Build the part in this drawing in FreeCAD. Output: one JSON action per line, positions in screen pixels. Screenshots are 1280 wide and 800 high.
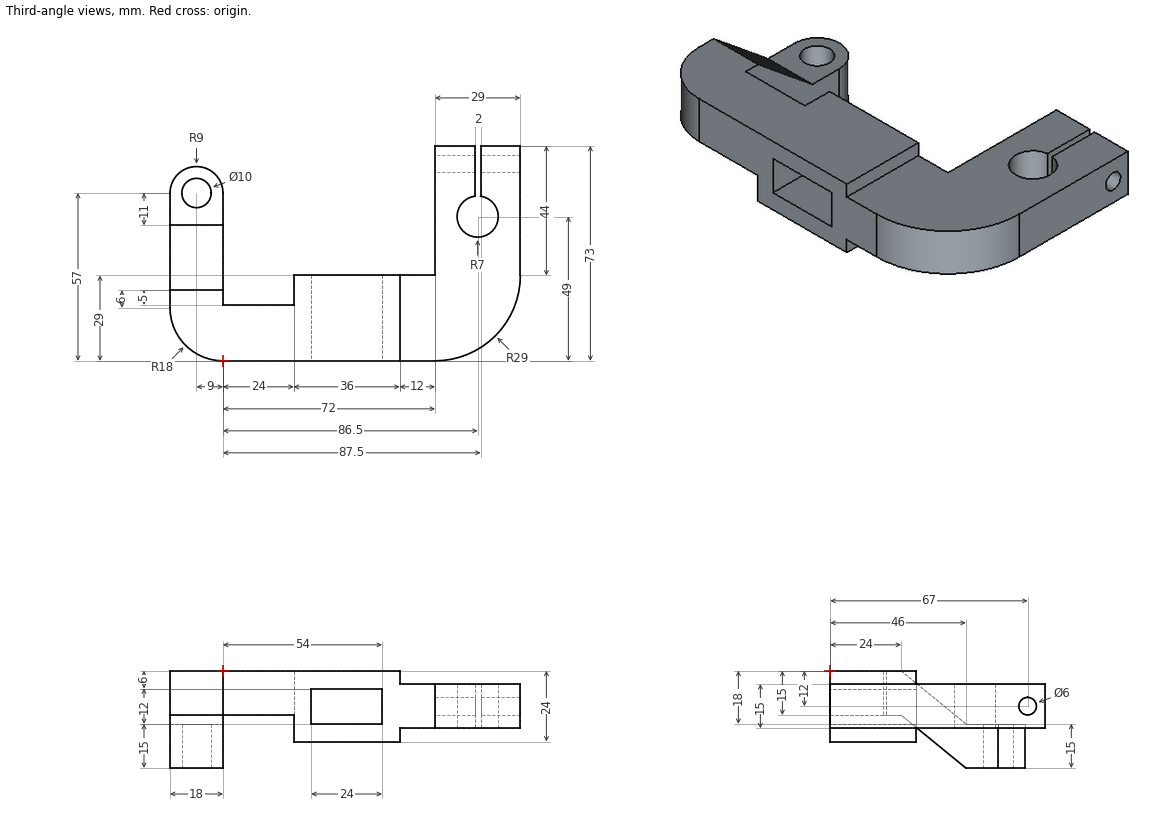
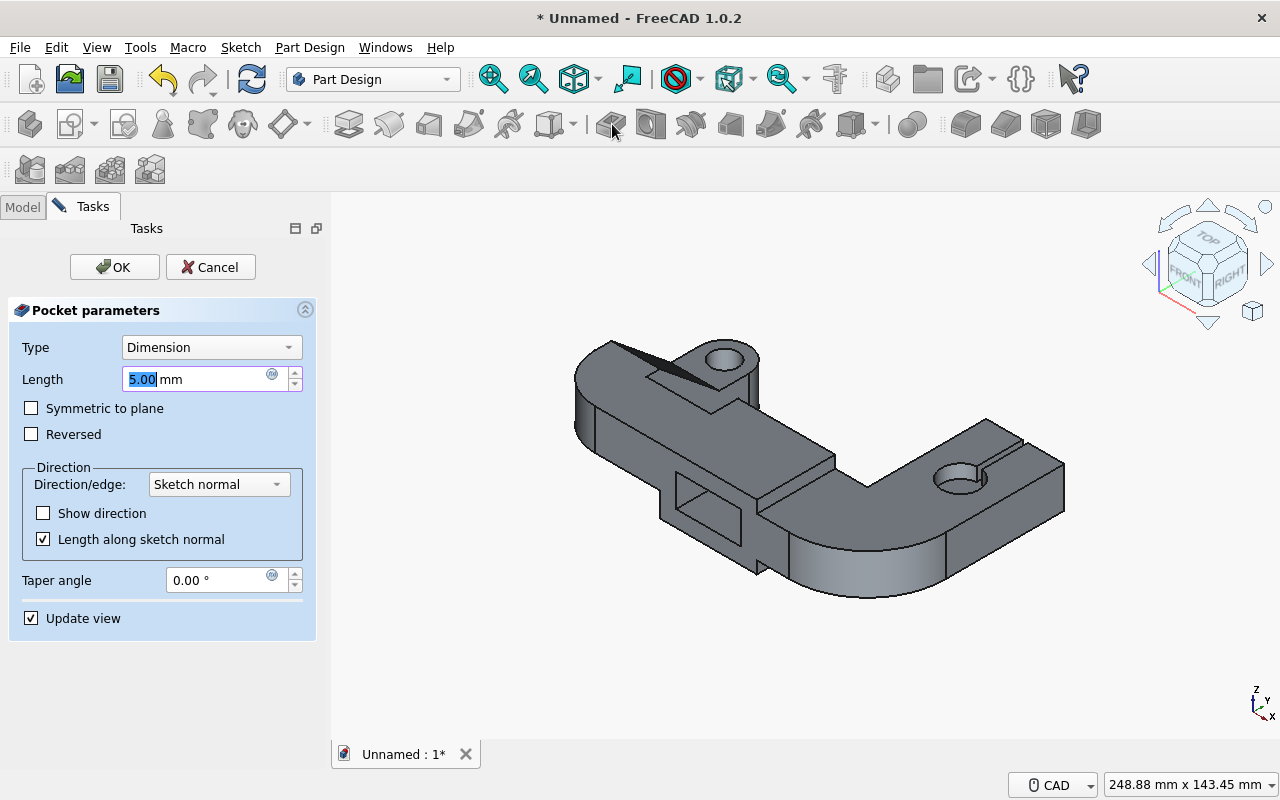
{"action": "type", "text": "15"}
{"action": "key", "text": "Tab"}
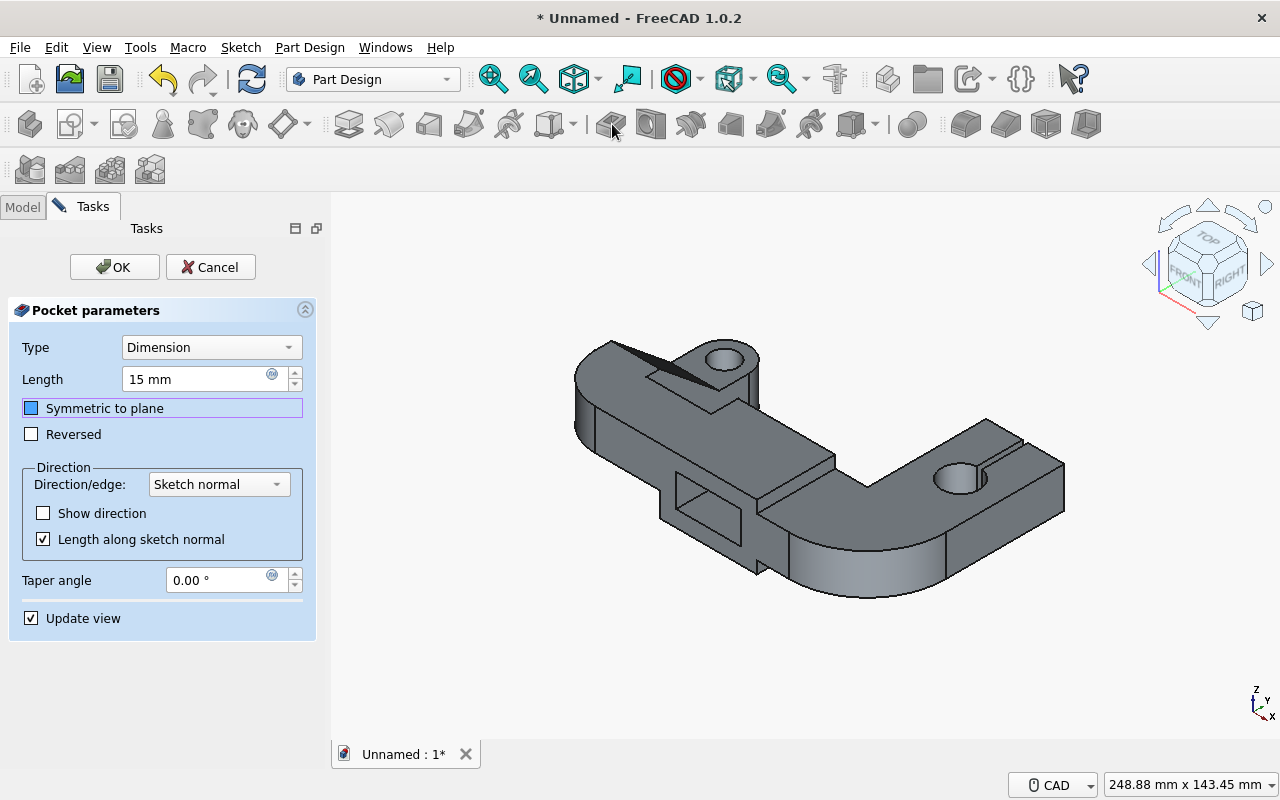
{"action": "left_click", "coordinate": [115, 267]}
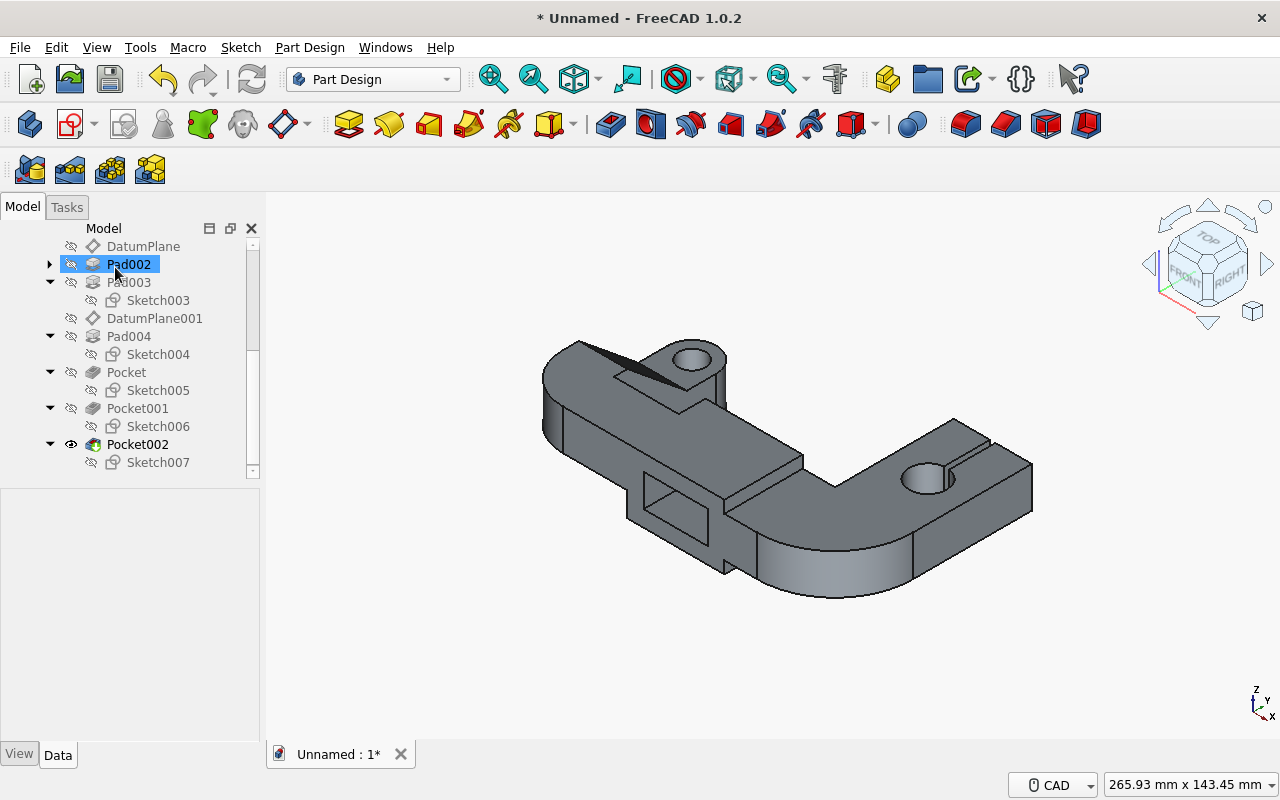
{"action": "key", "text": "6"}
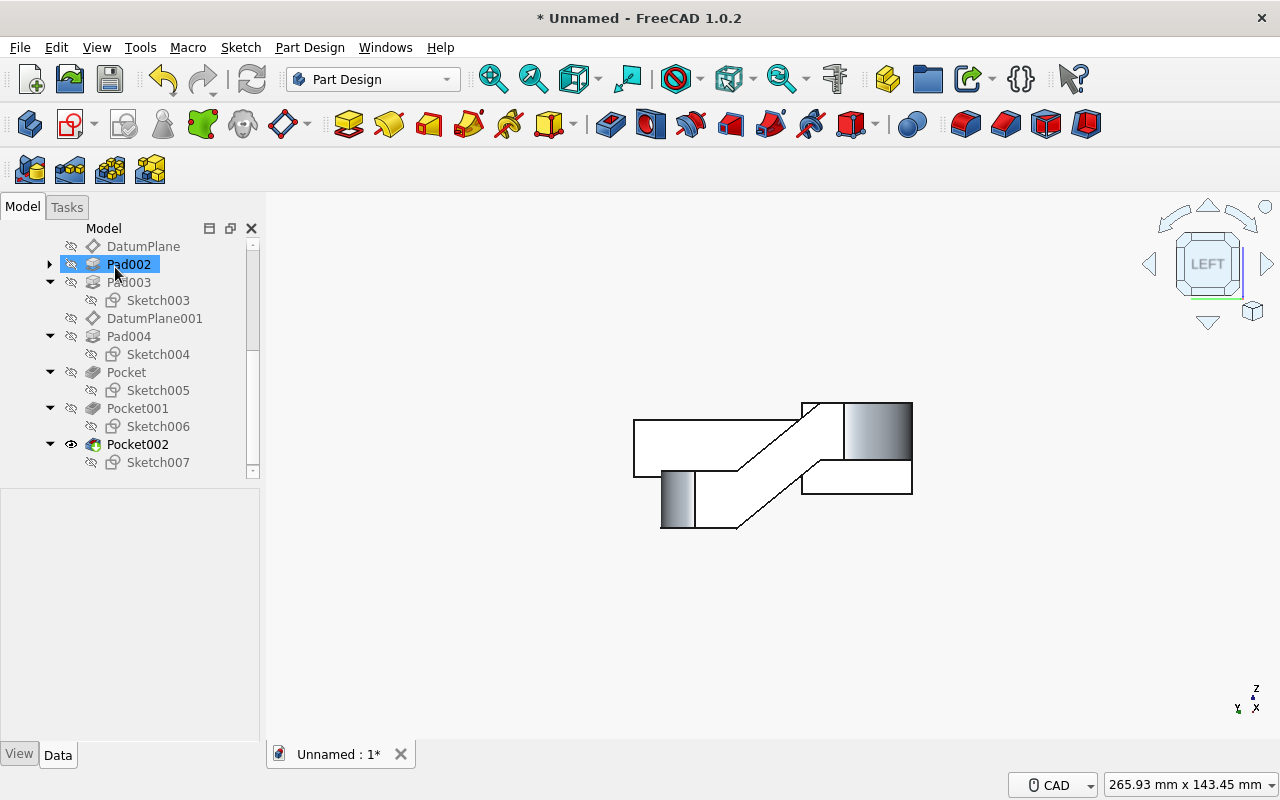
{"action": "left_click", "coordinate": [494, 80]}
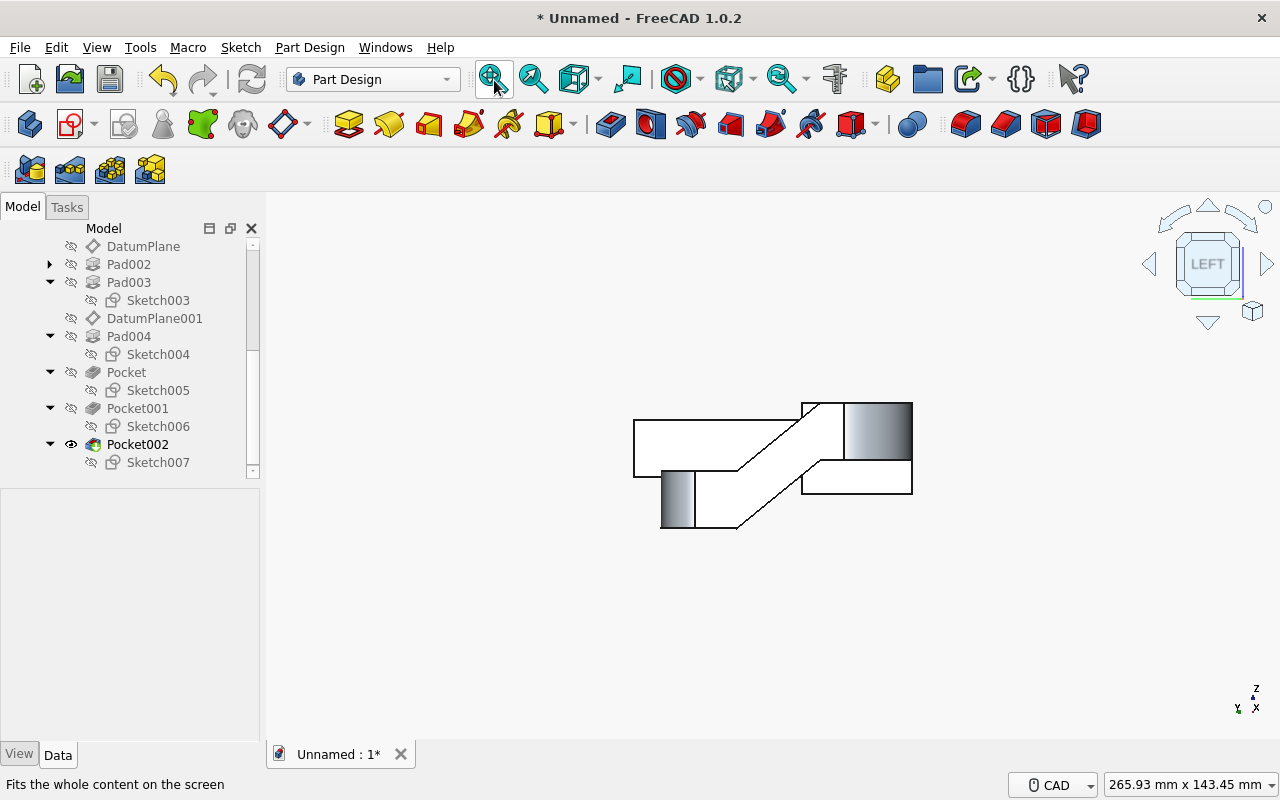
{"action": "left_click", "coordinate": [670, 447]}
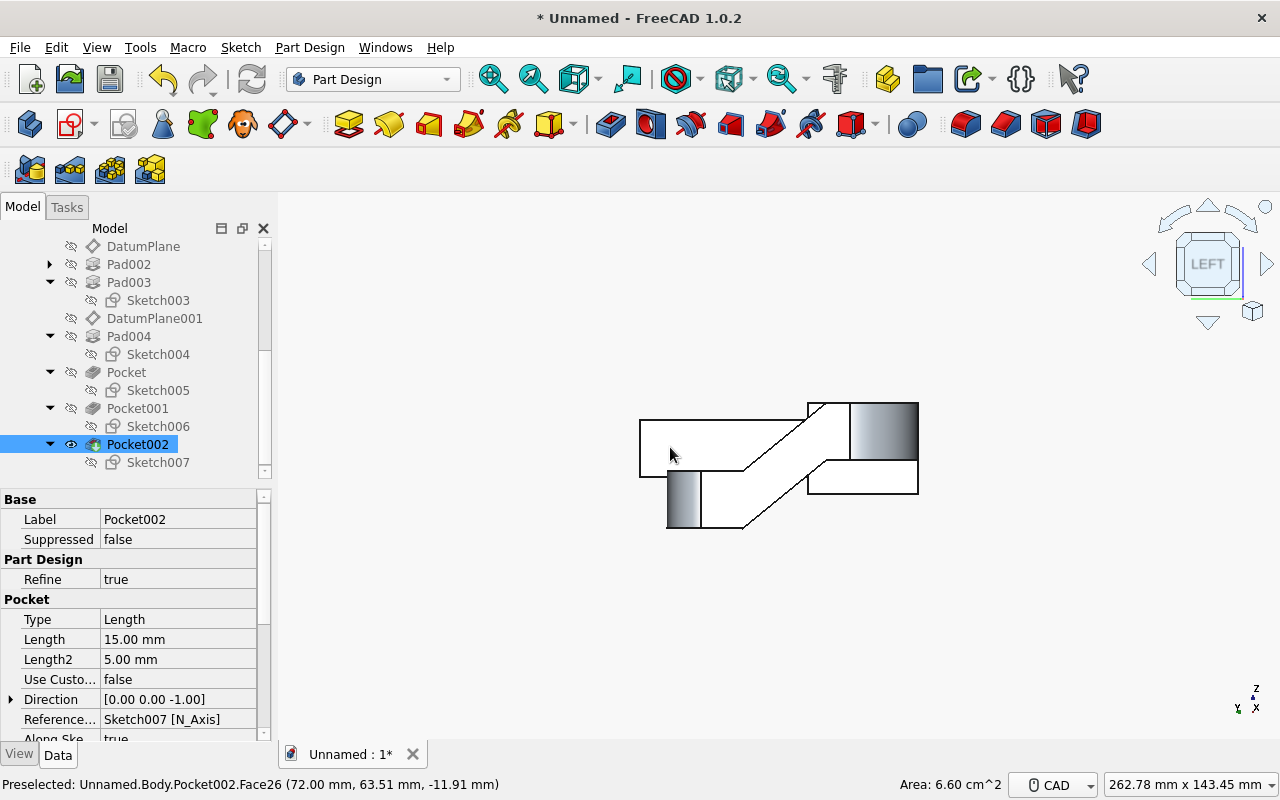
{"action": "left_click", "coordinate": [70, 124]}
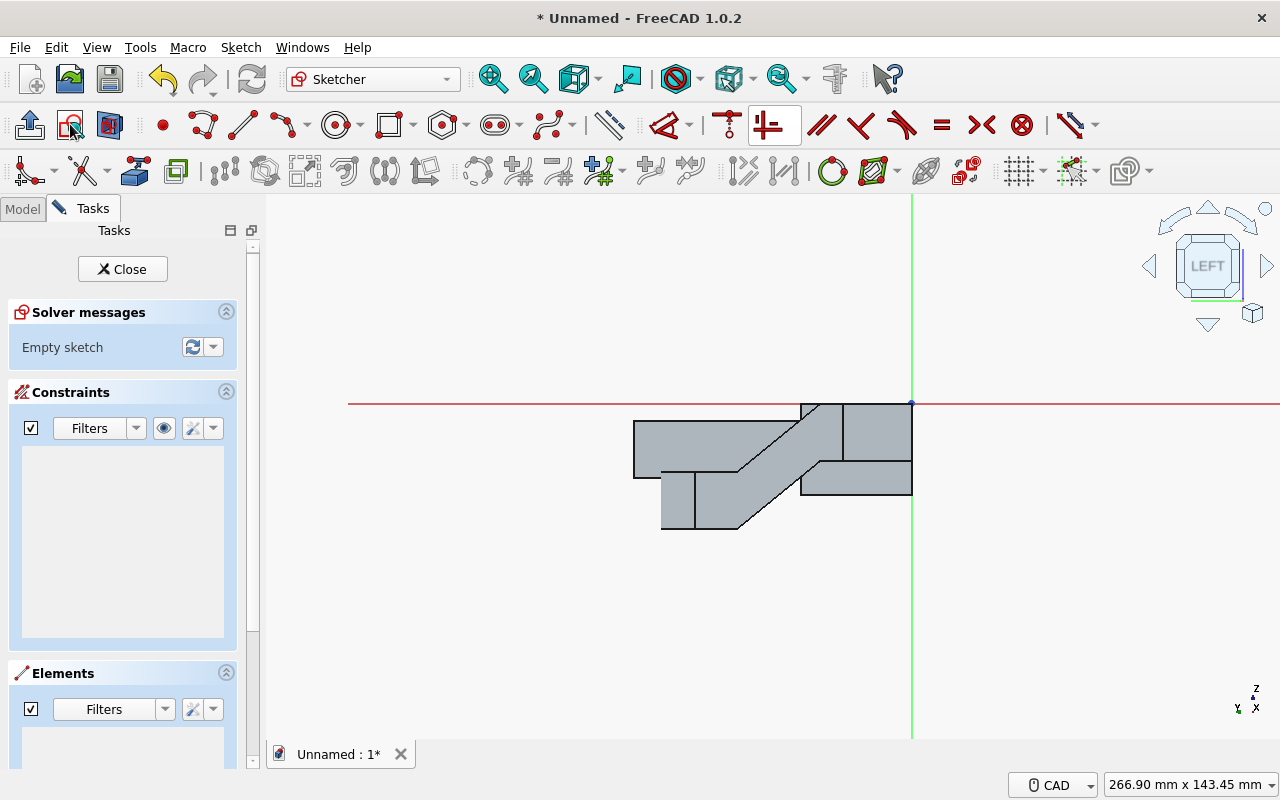
{"action": "scroll", "coordinate": [654, 448], "scroll_direction": "up", "scroll_amount": 14}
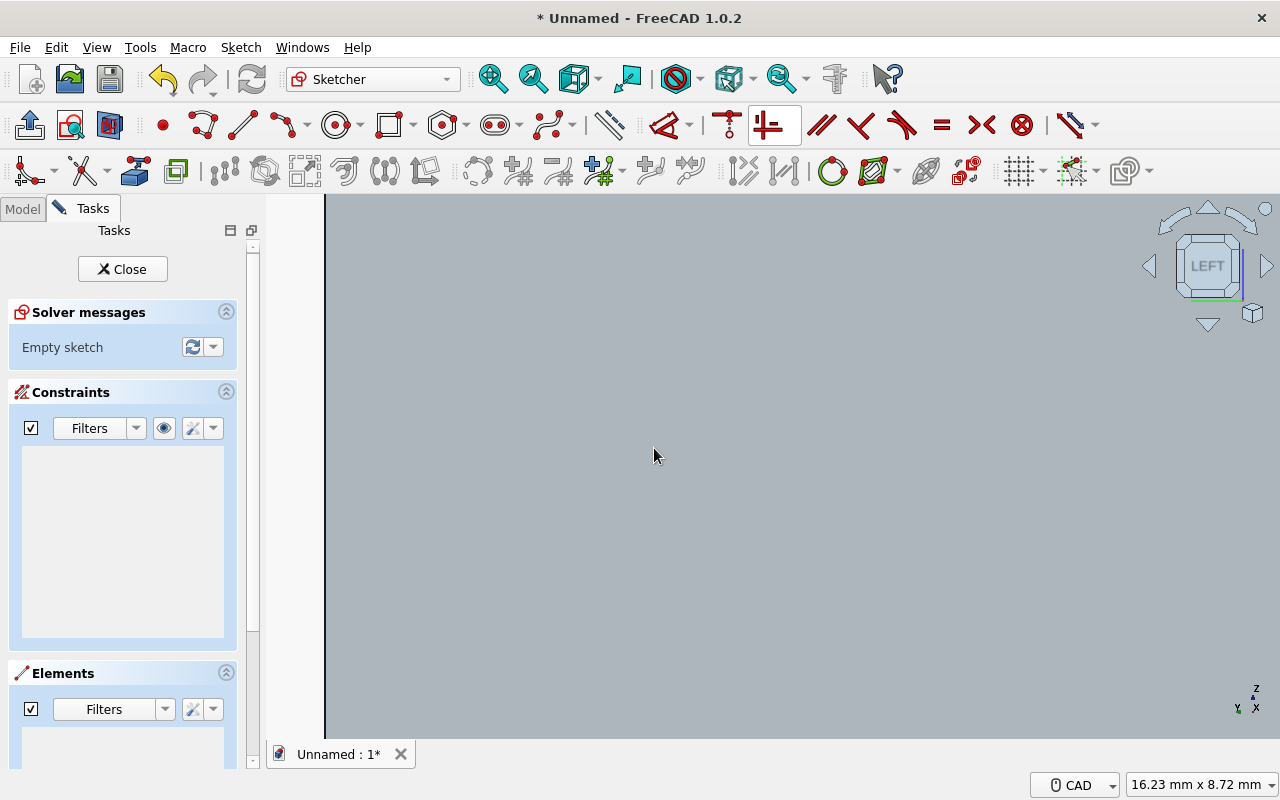
{"action": "left_click", "coordinate": [336, 126]}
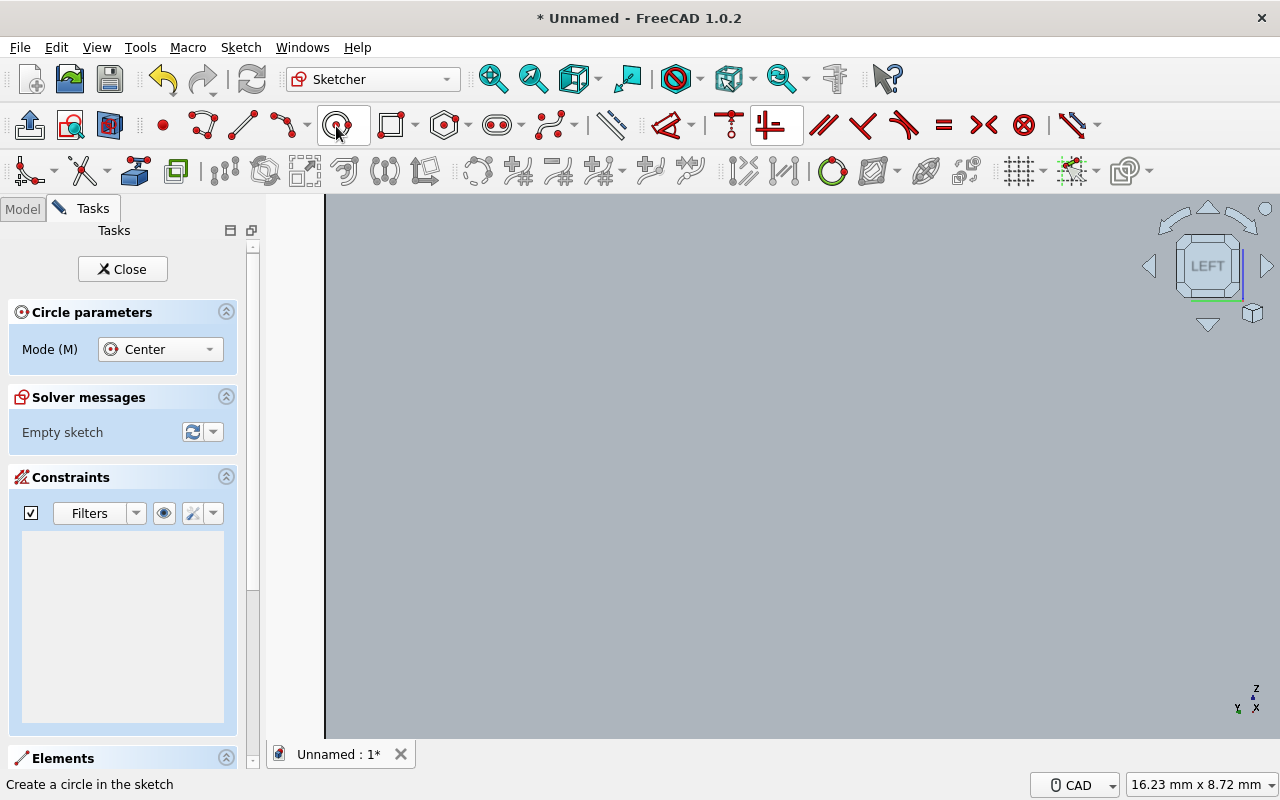
{"action": "left_click", "coordinate": [699, 464]}
{"action": "mouse_move", "coordinate": [832, 331]}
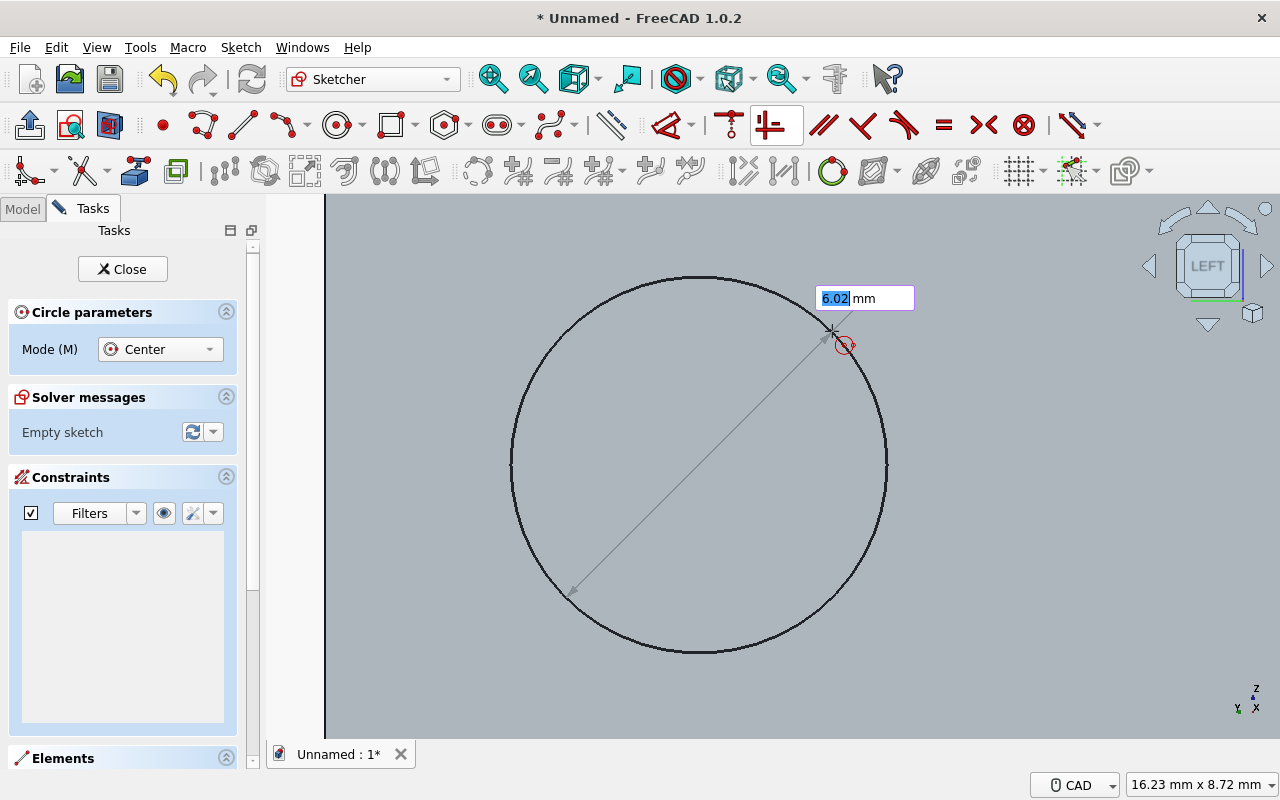
{"action": "type", "text": "6"}
{"action": "key", "text": "Return"}
{"action": "key", "text": "Escape"}